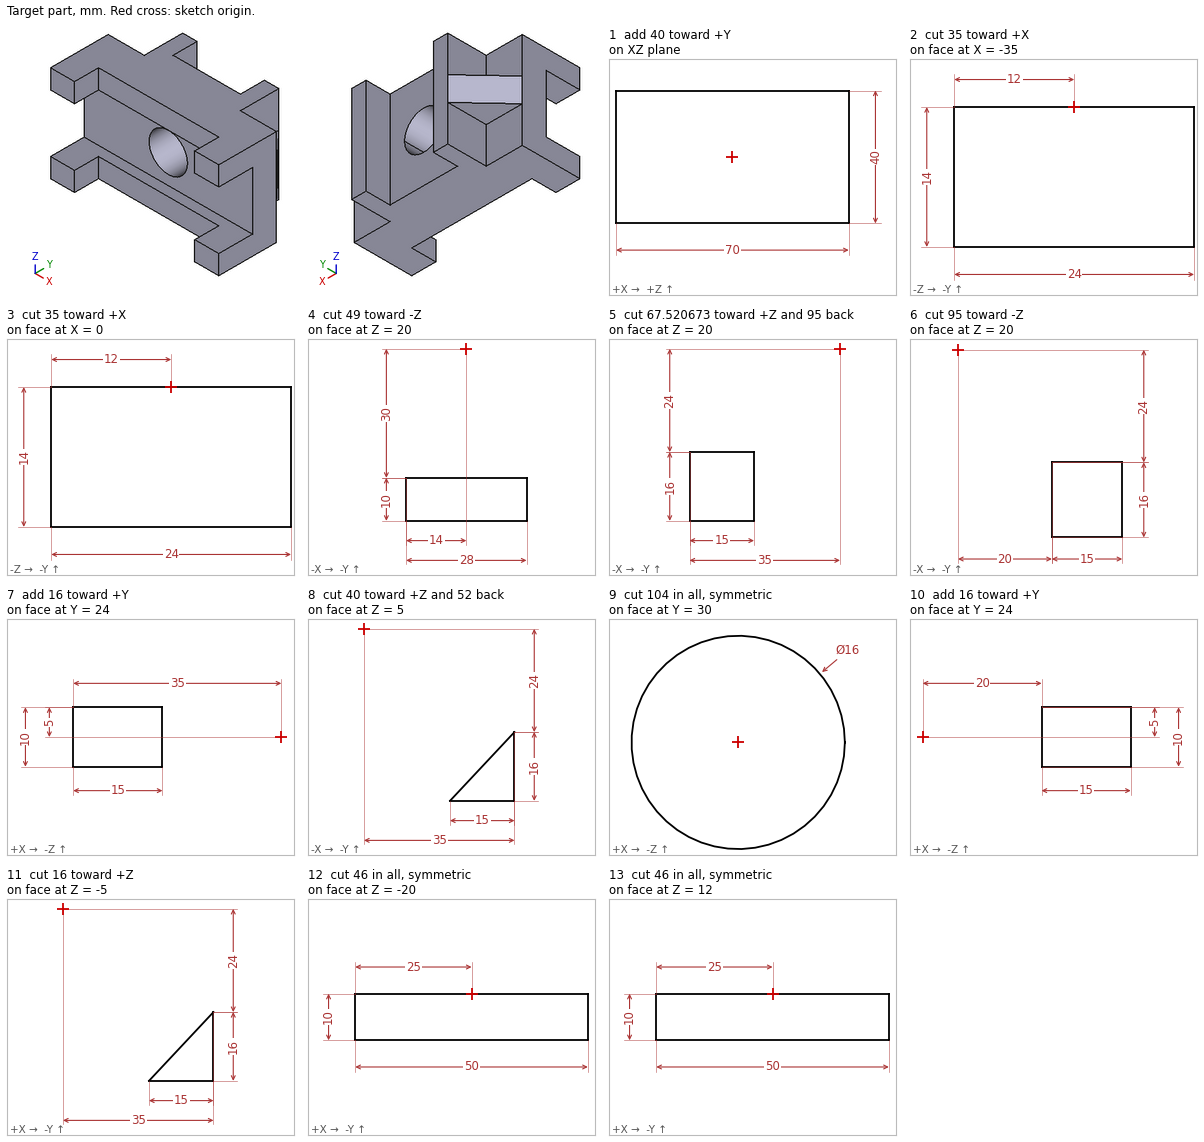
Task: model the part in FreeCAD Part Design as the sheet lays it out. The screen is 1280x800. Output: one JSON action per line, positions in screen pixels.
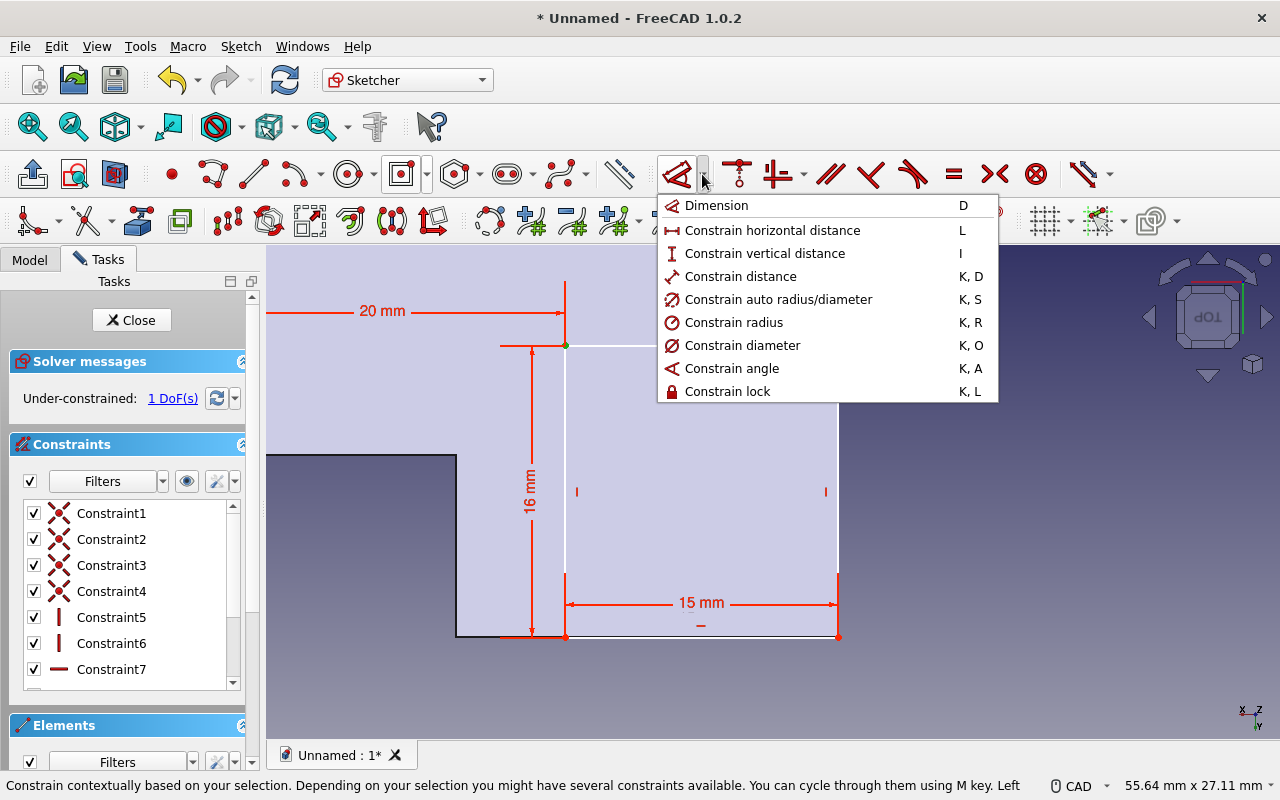
{"action": "left_click", "coordinate": [828, 254]}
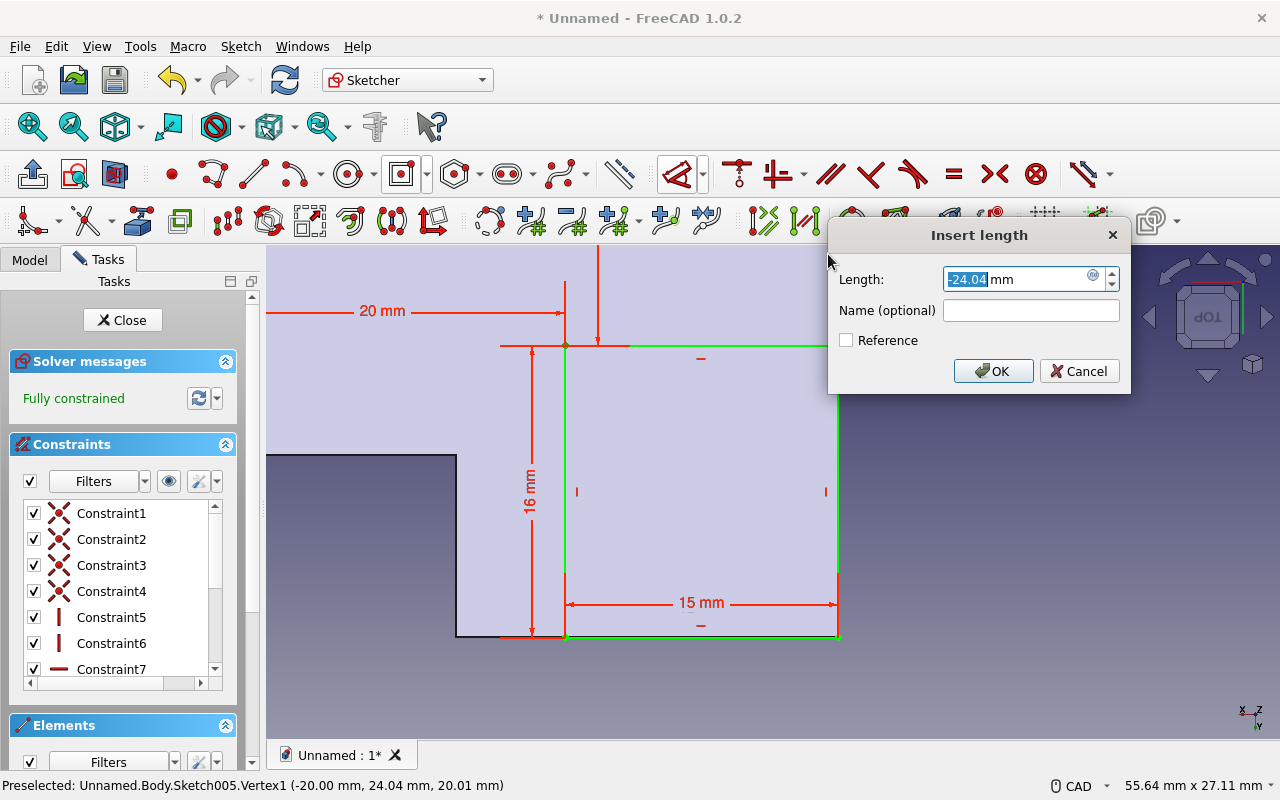
{"action": "type", "text": "-24"}
{"action": "key", "text": "Return"}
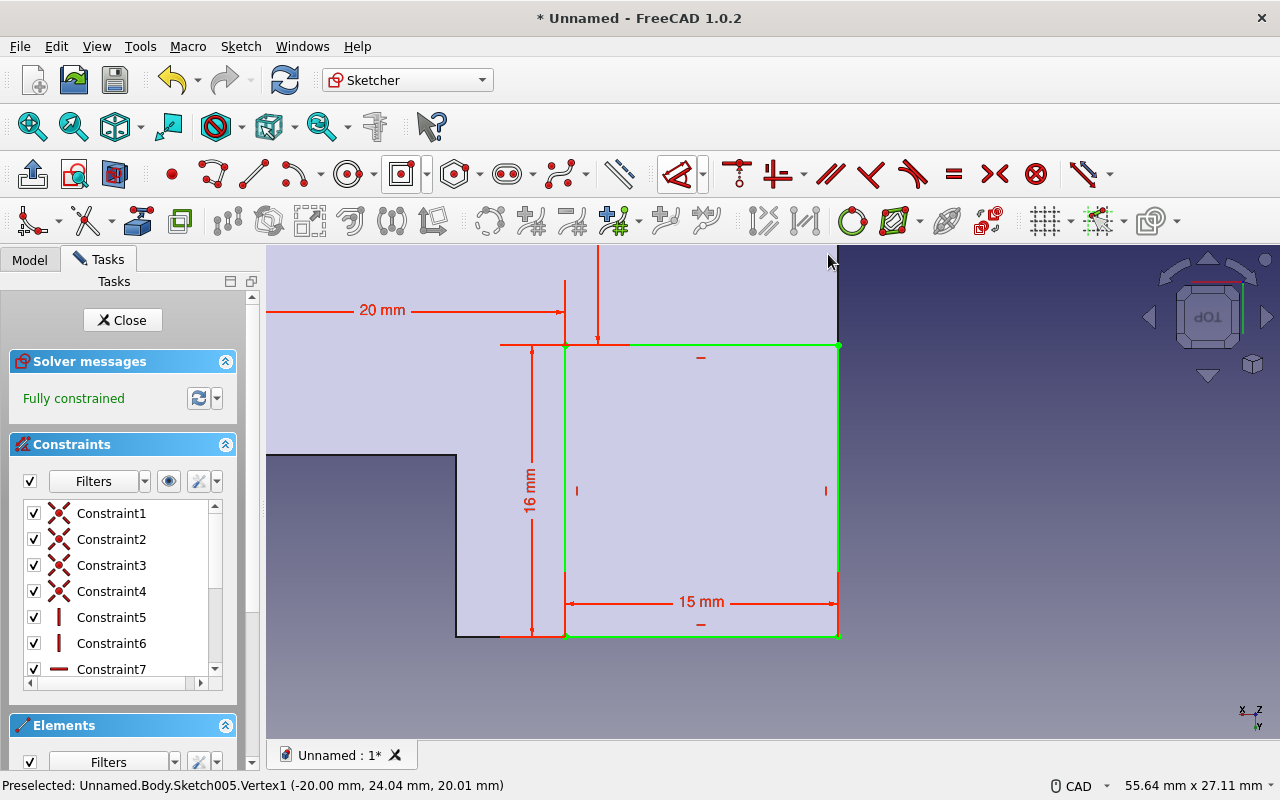
{"action": "left_click", "coordinate": [123, 320]}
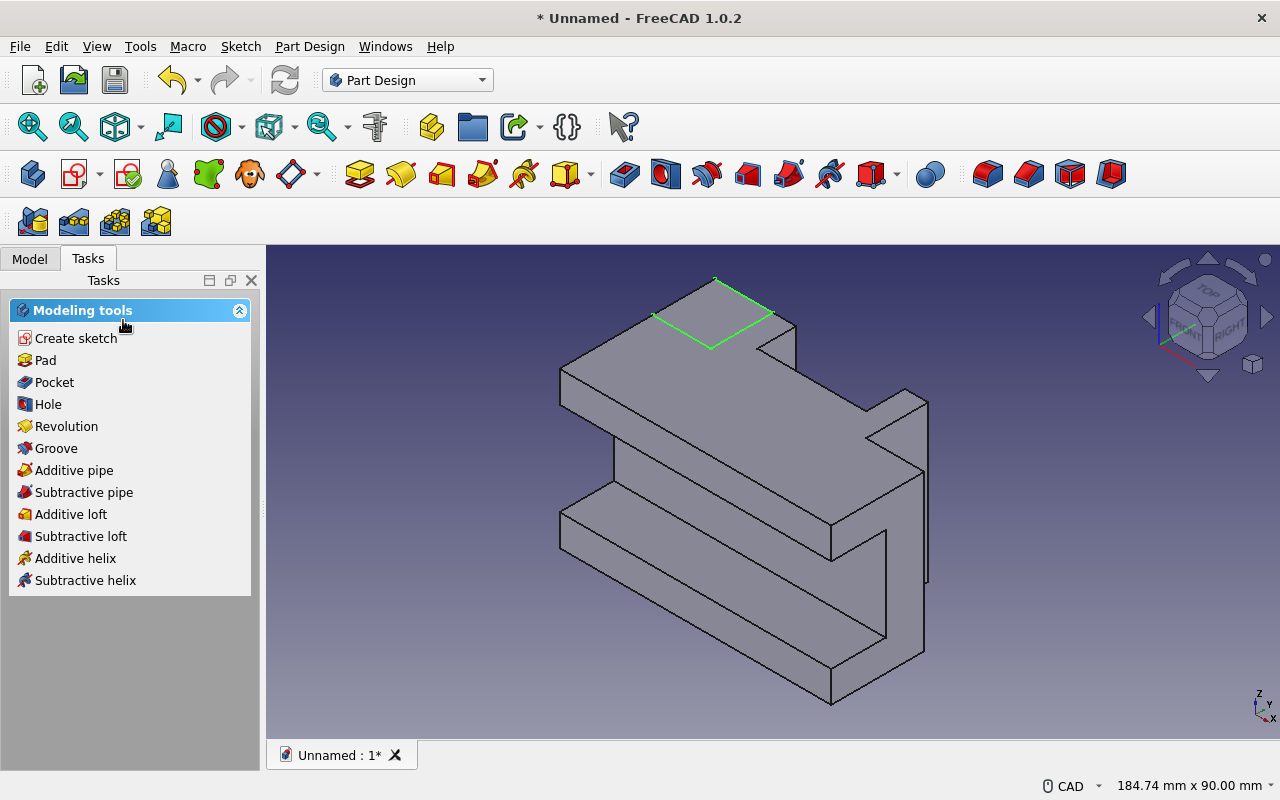
{"action": "left_click", "coordinate": [625, 174]}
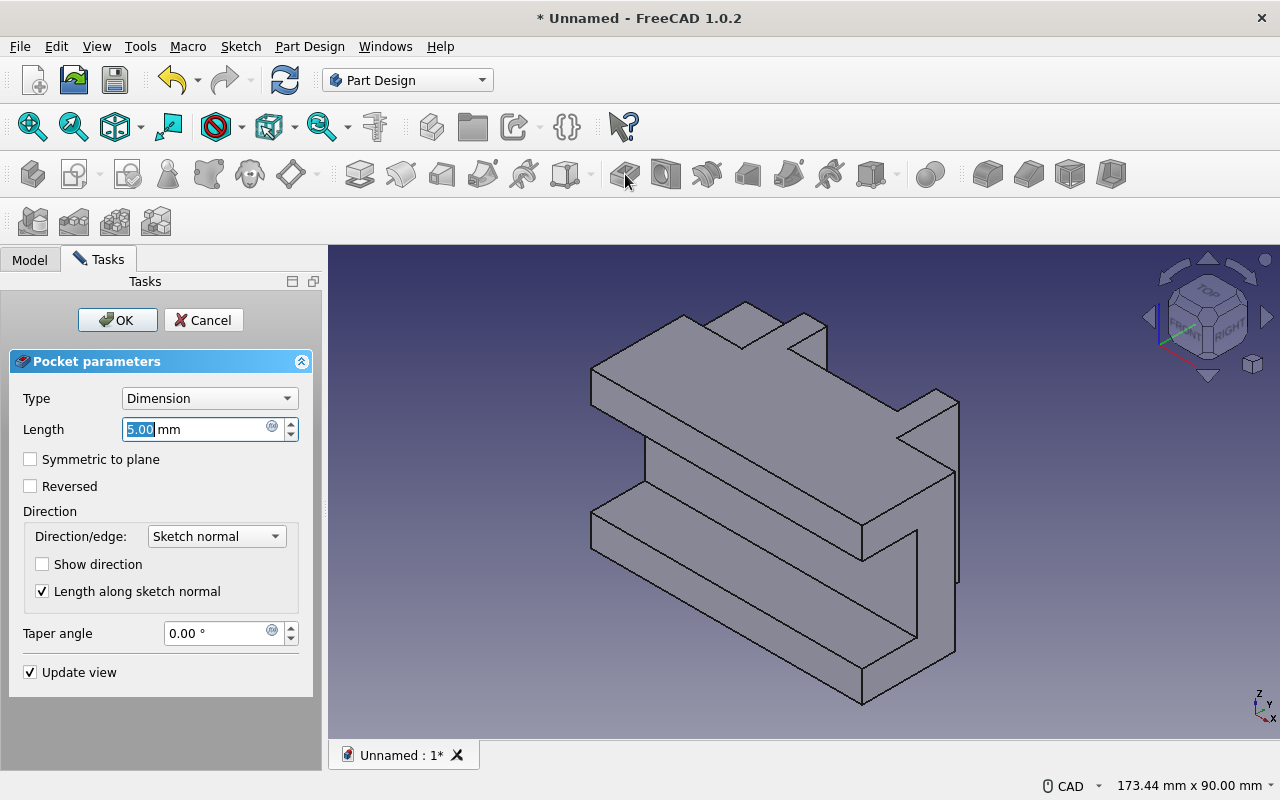
{"action": "type", "text": "95"}
{"action": "key", "text": "Tab"}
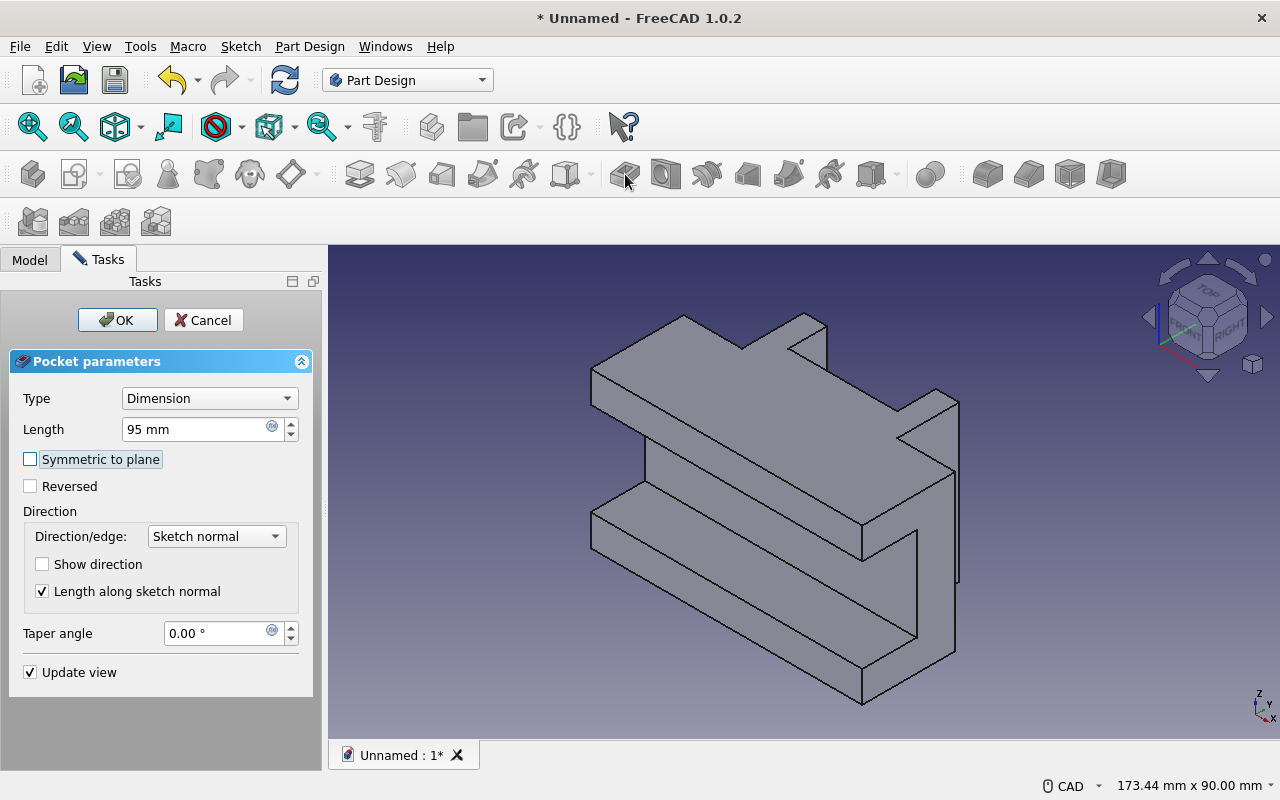
{"action": "left_click", "coordinate": [118, 320]}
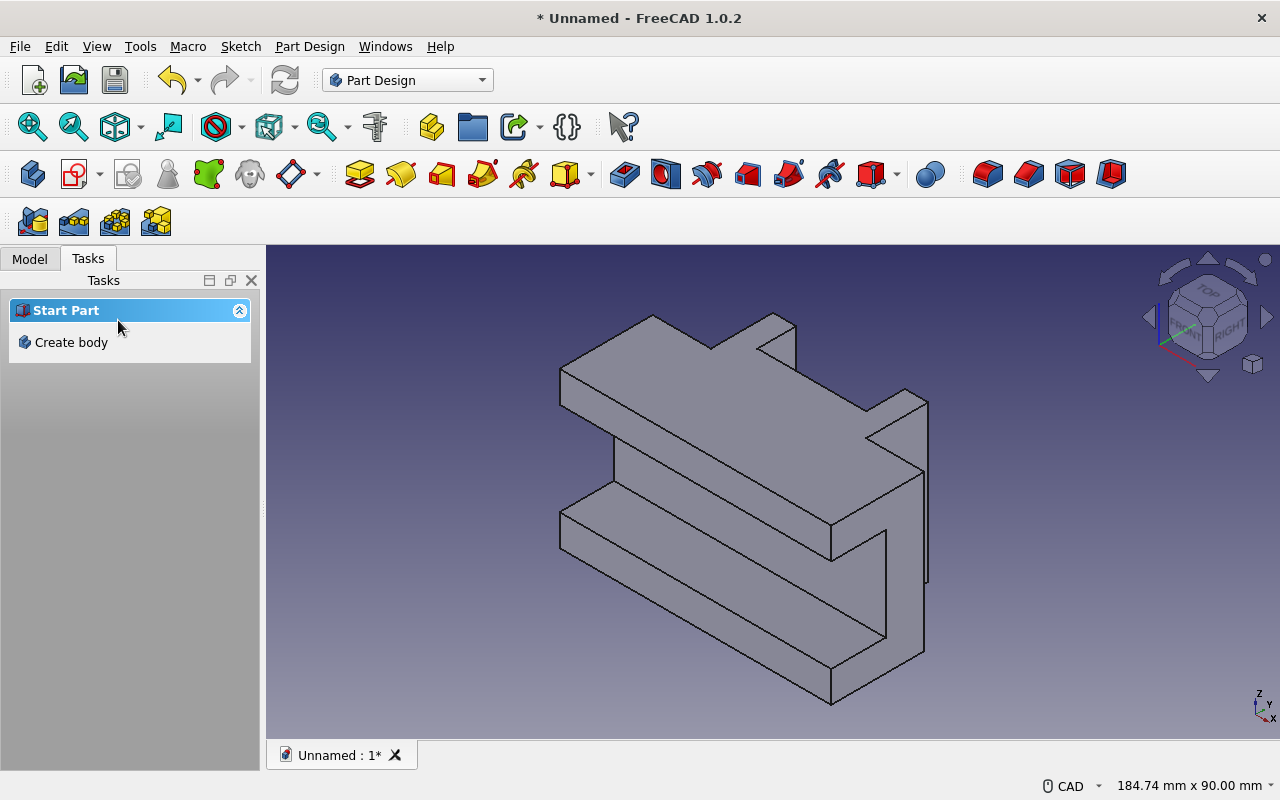
{"action": "key", "text": "4"}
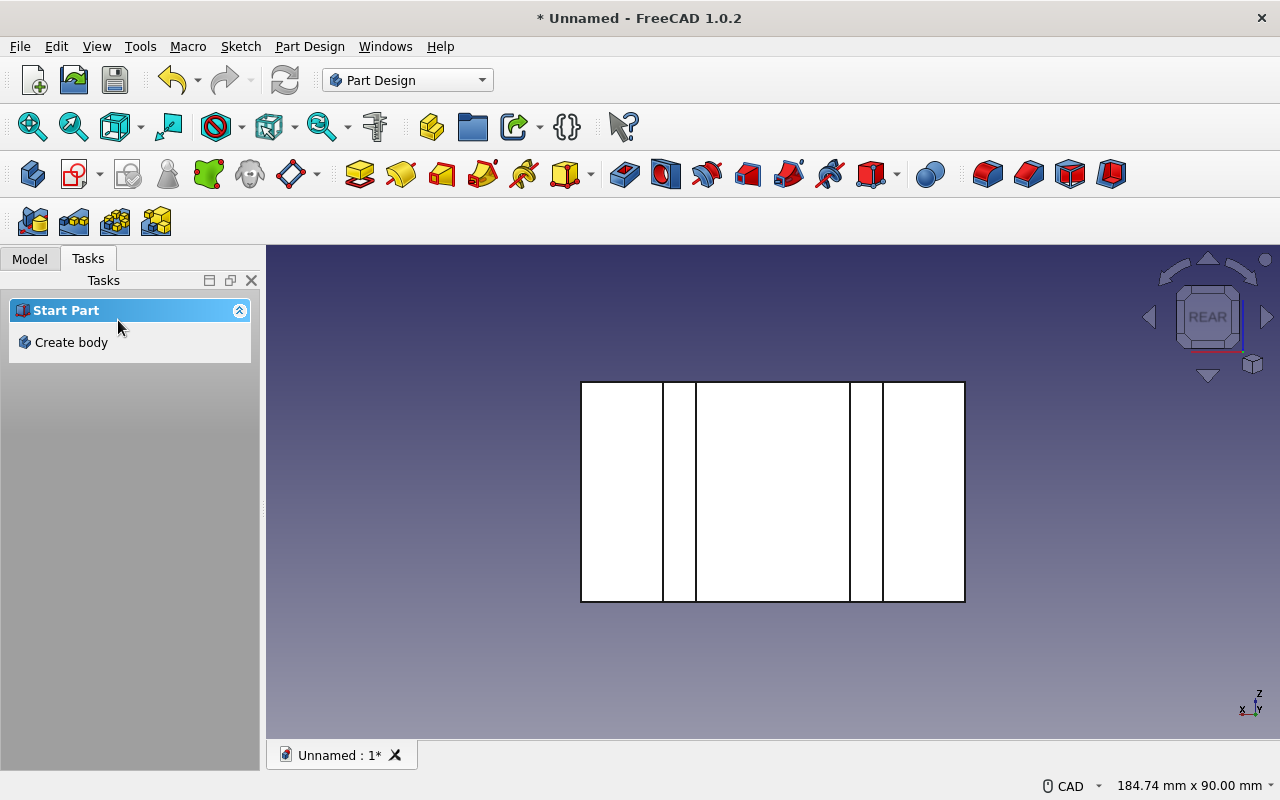
{"action": "key", "text": "v f"}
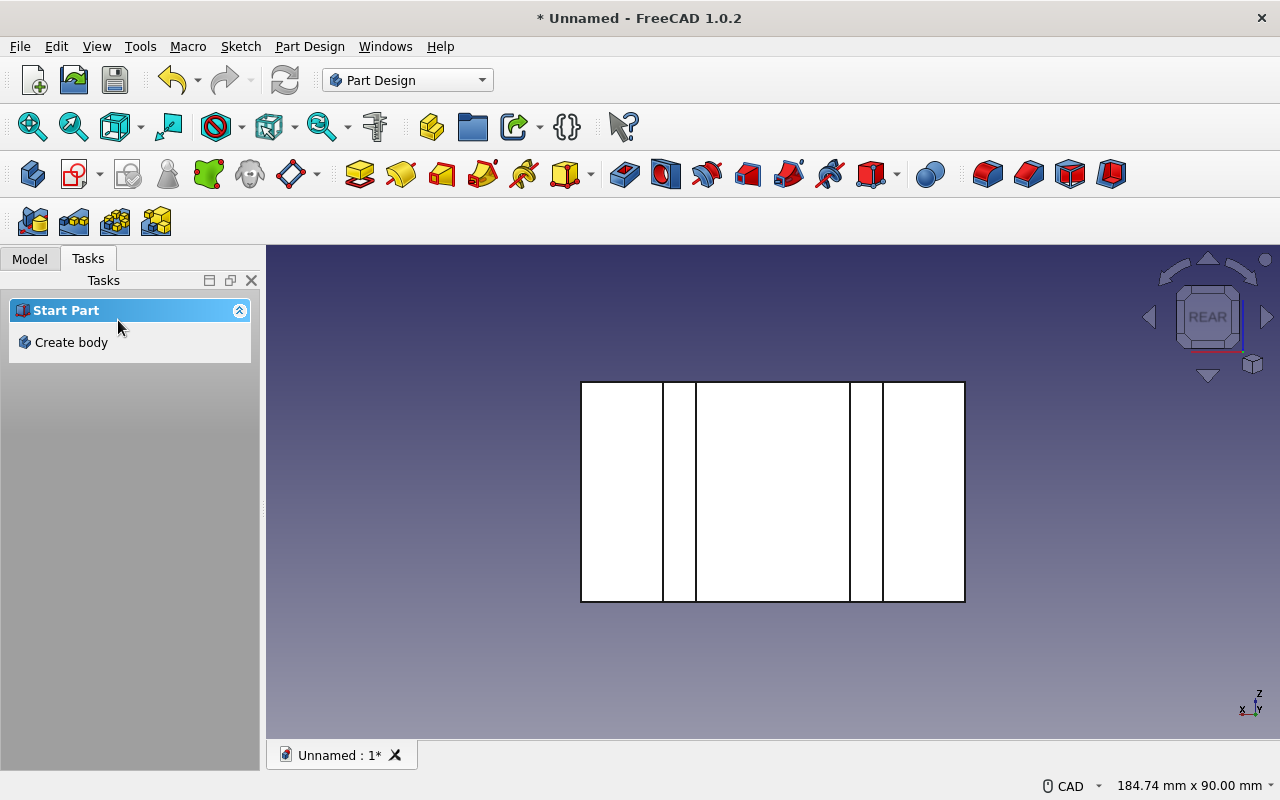
{"action": "left_click", "coordinate": [622, 460]}